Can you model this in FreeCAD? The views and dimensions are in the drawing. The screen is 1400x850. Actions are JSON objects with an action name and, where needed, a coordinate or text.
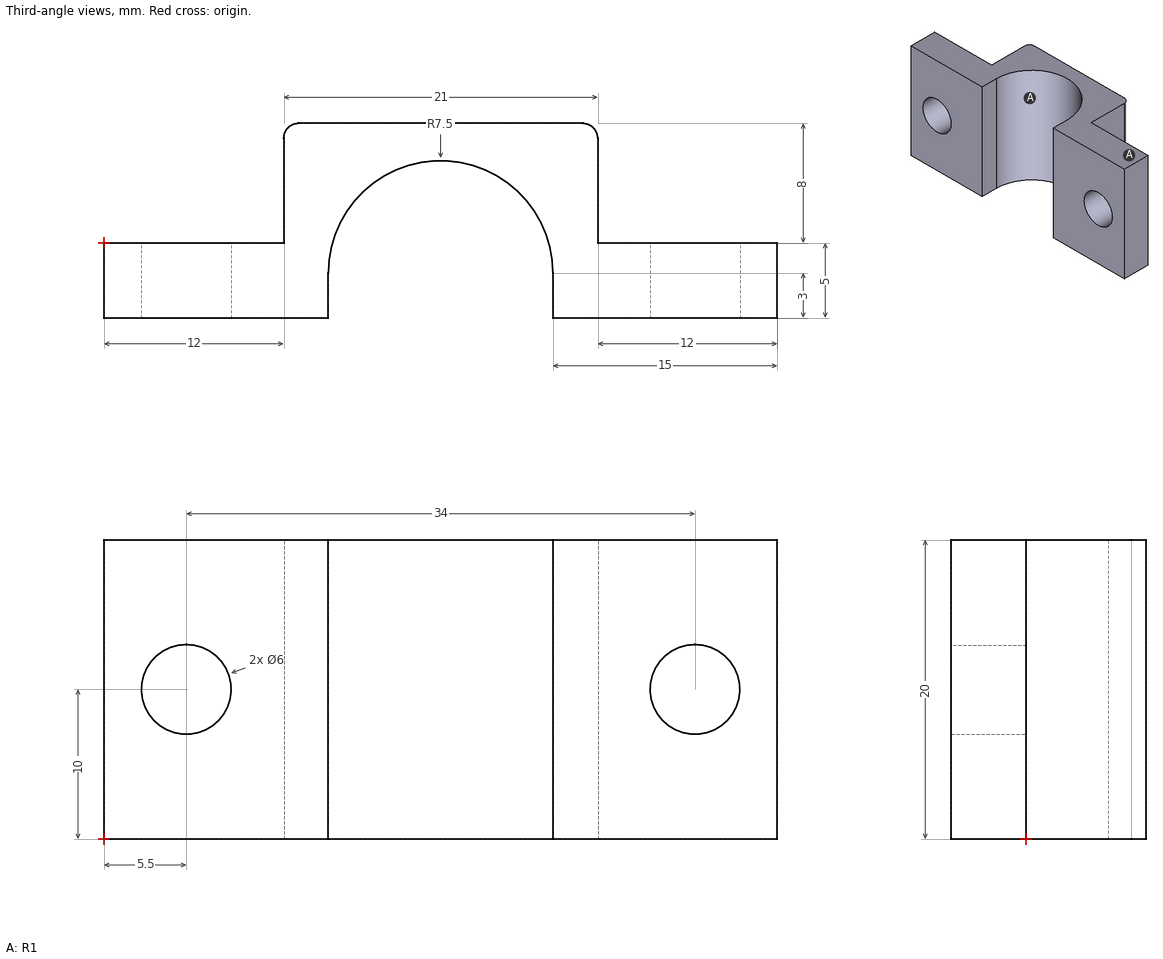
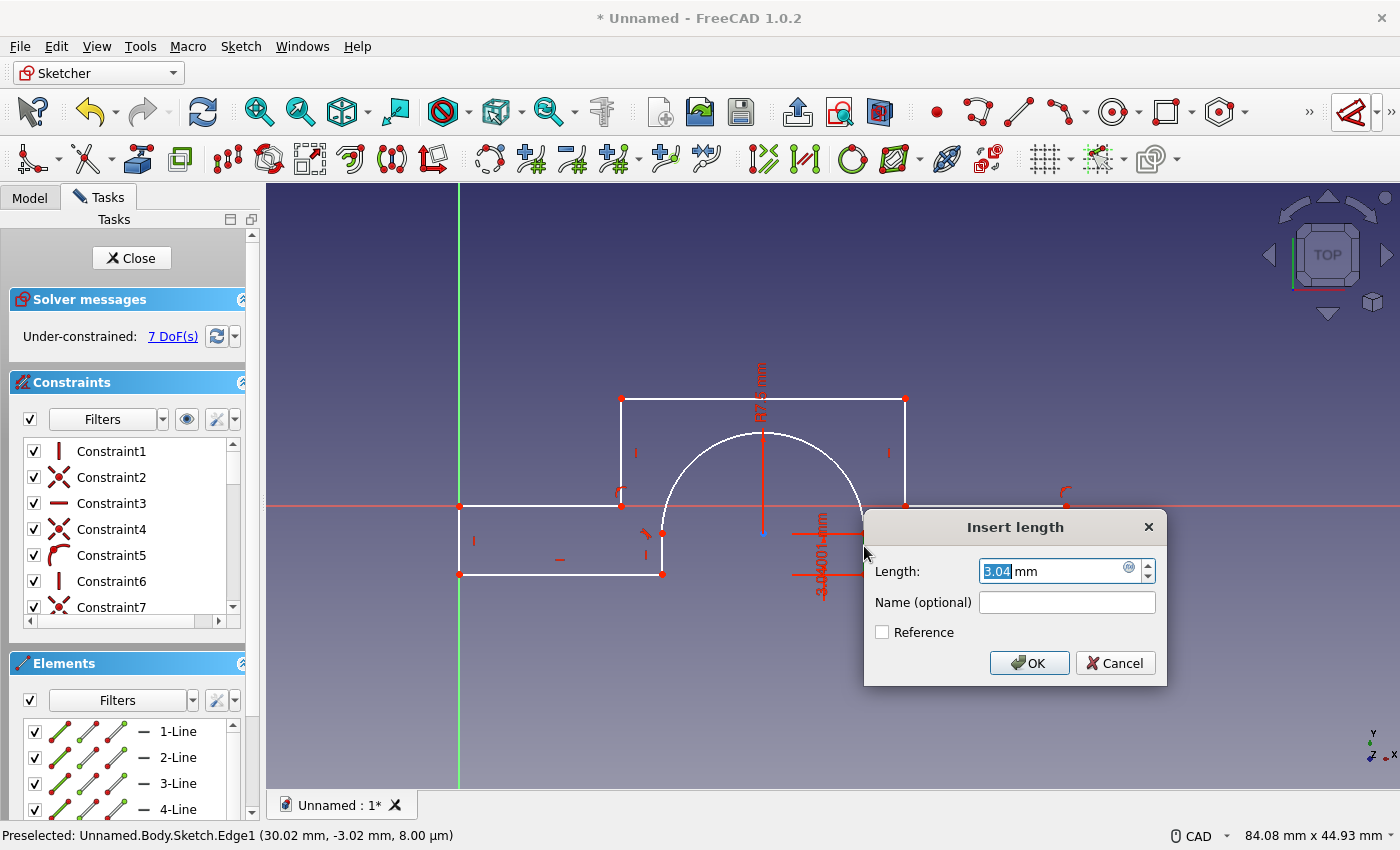
{"action": "type", "text": "3"}
{"action": "key", "text": "Return"}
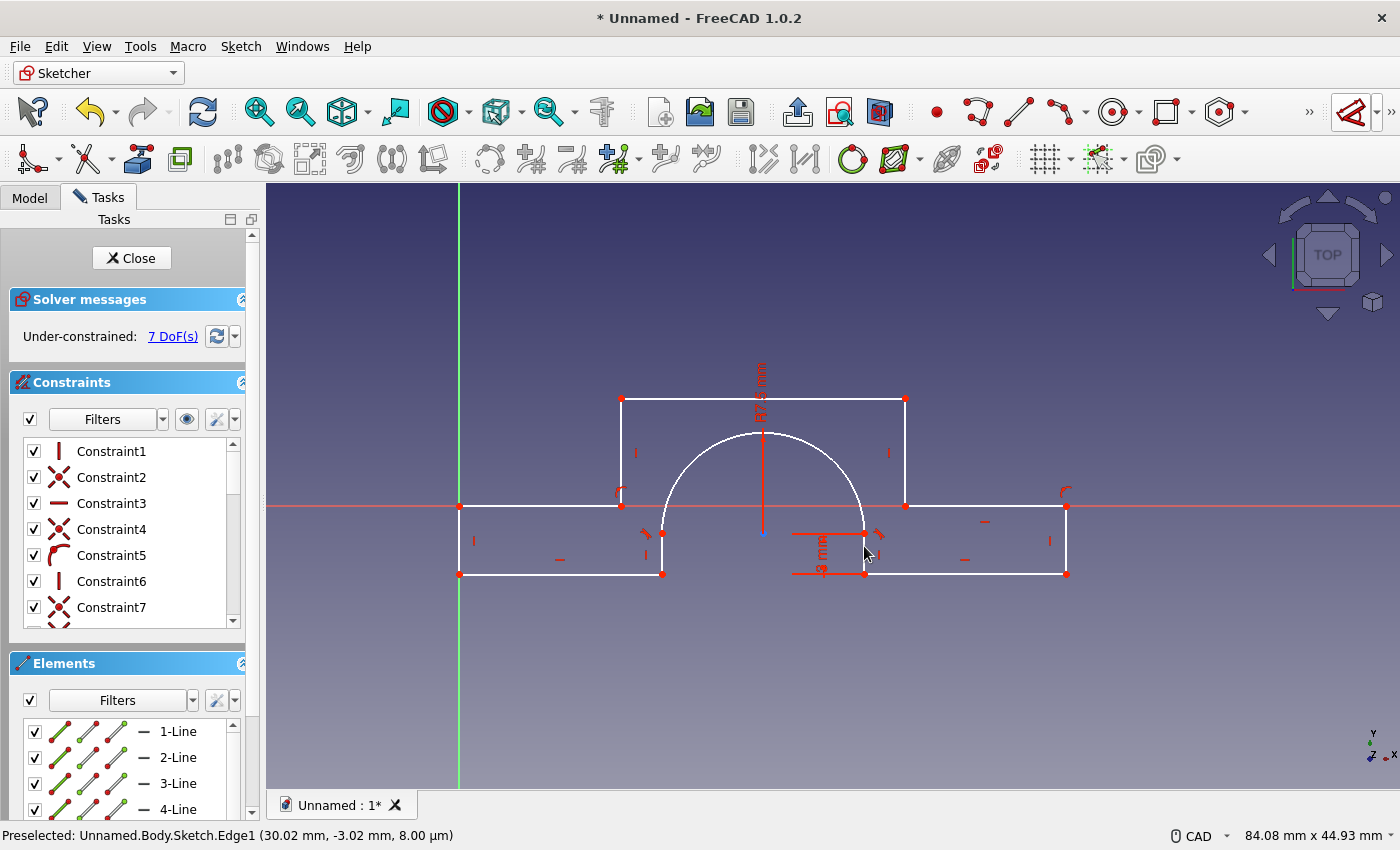
{"action": "left_click", "coordinate": [1066, 554]}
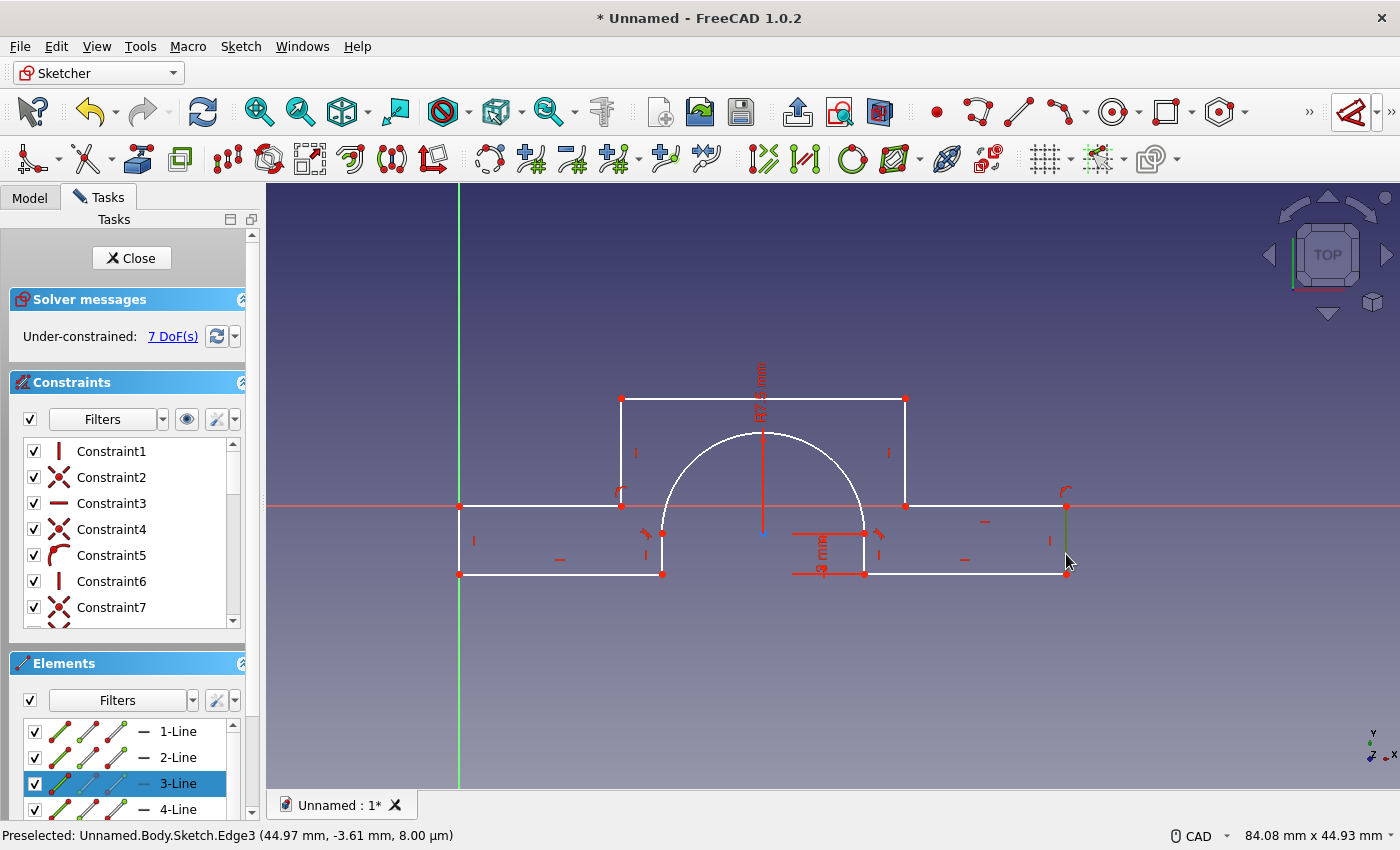
{"action": "key", "text": "i"}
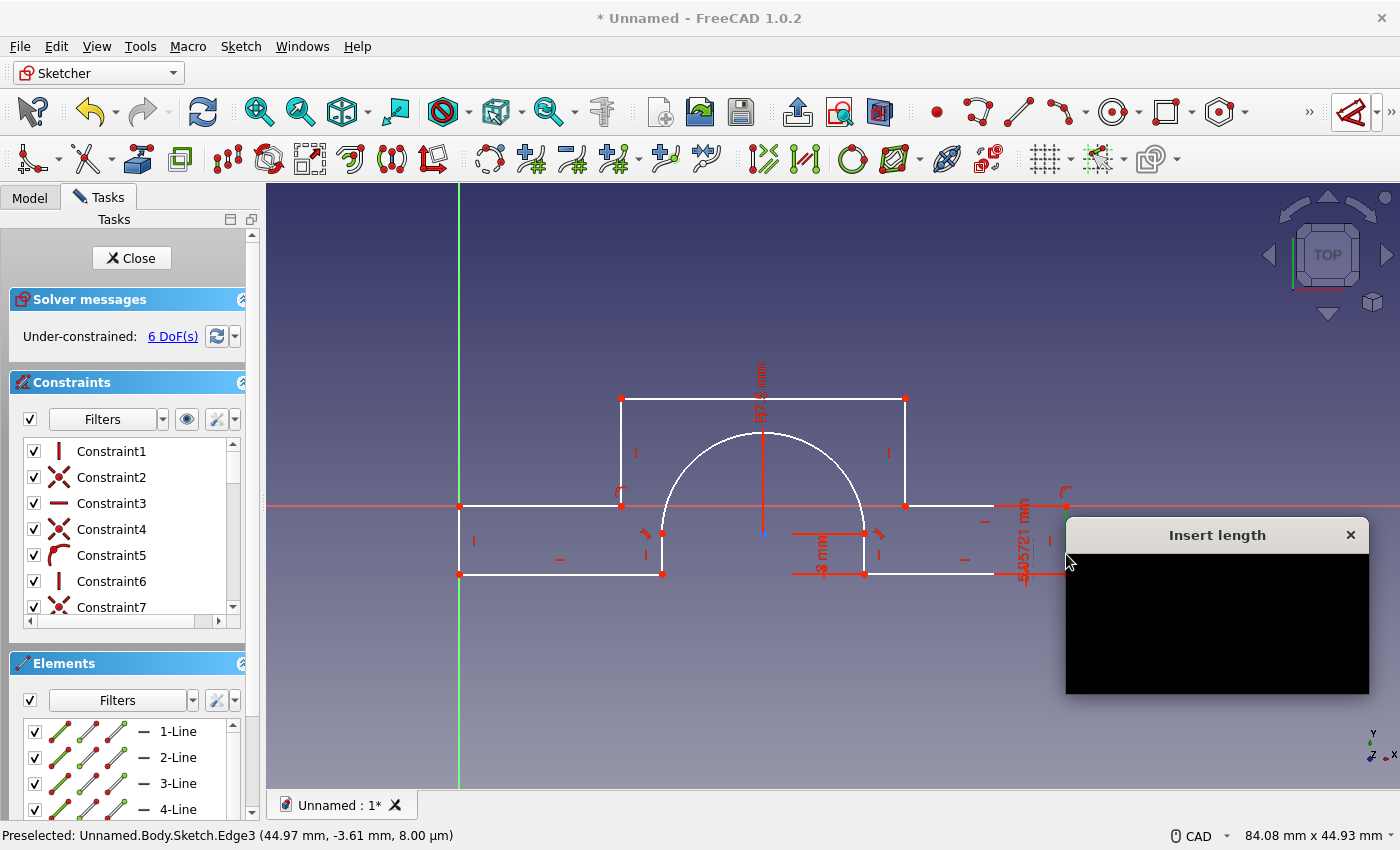
{"action": "type", "text": "5"}
{"action": "key", "text": "Return"}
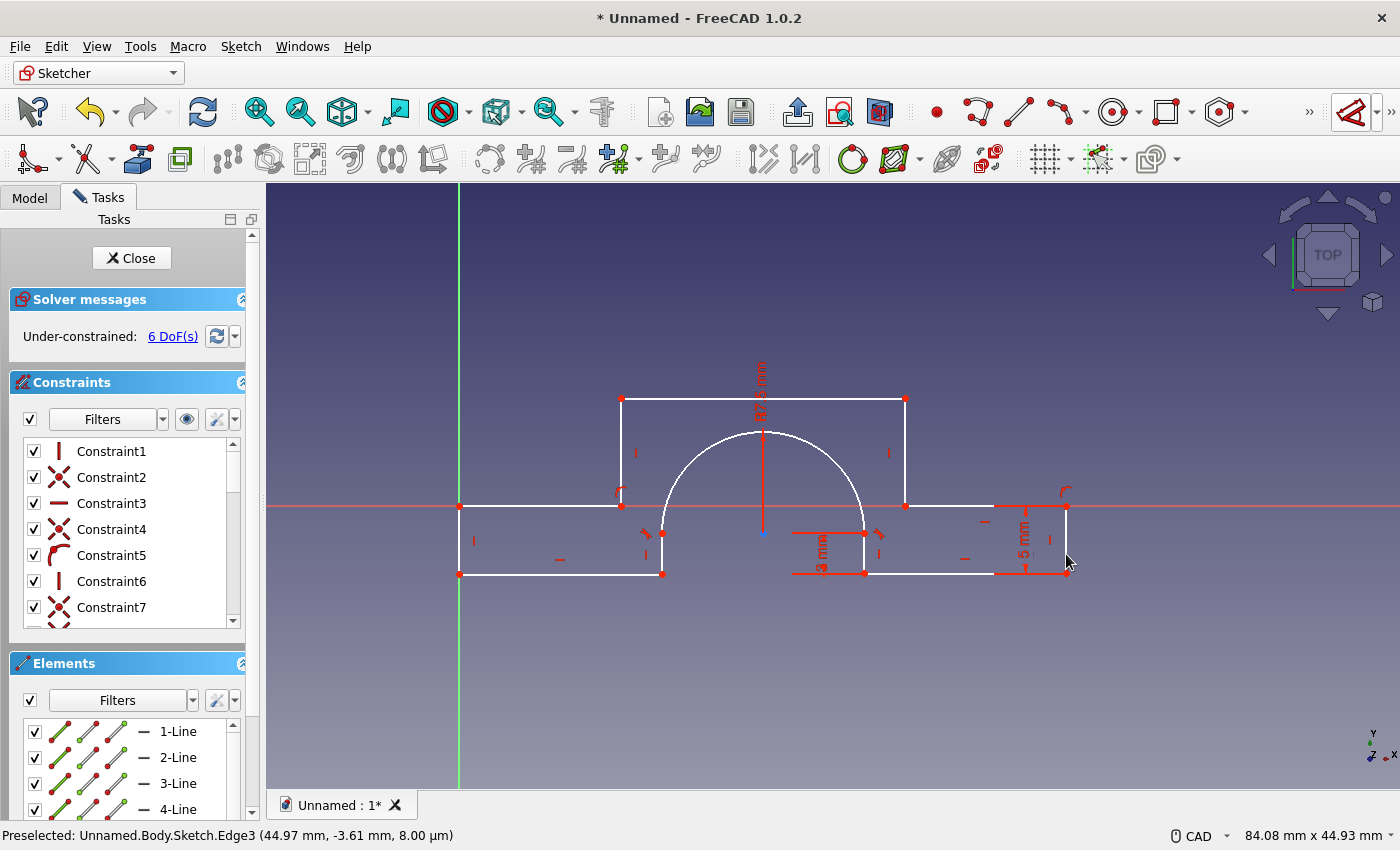
{"action": "left_click", "coordinate": [905, 474]}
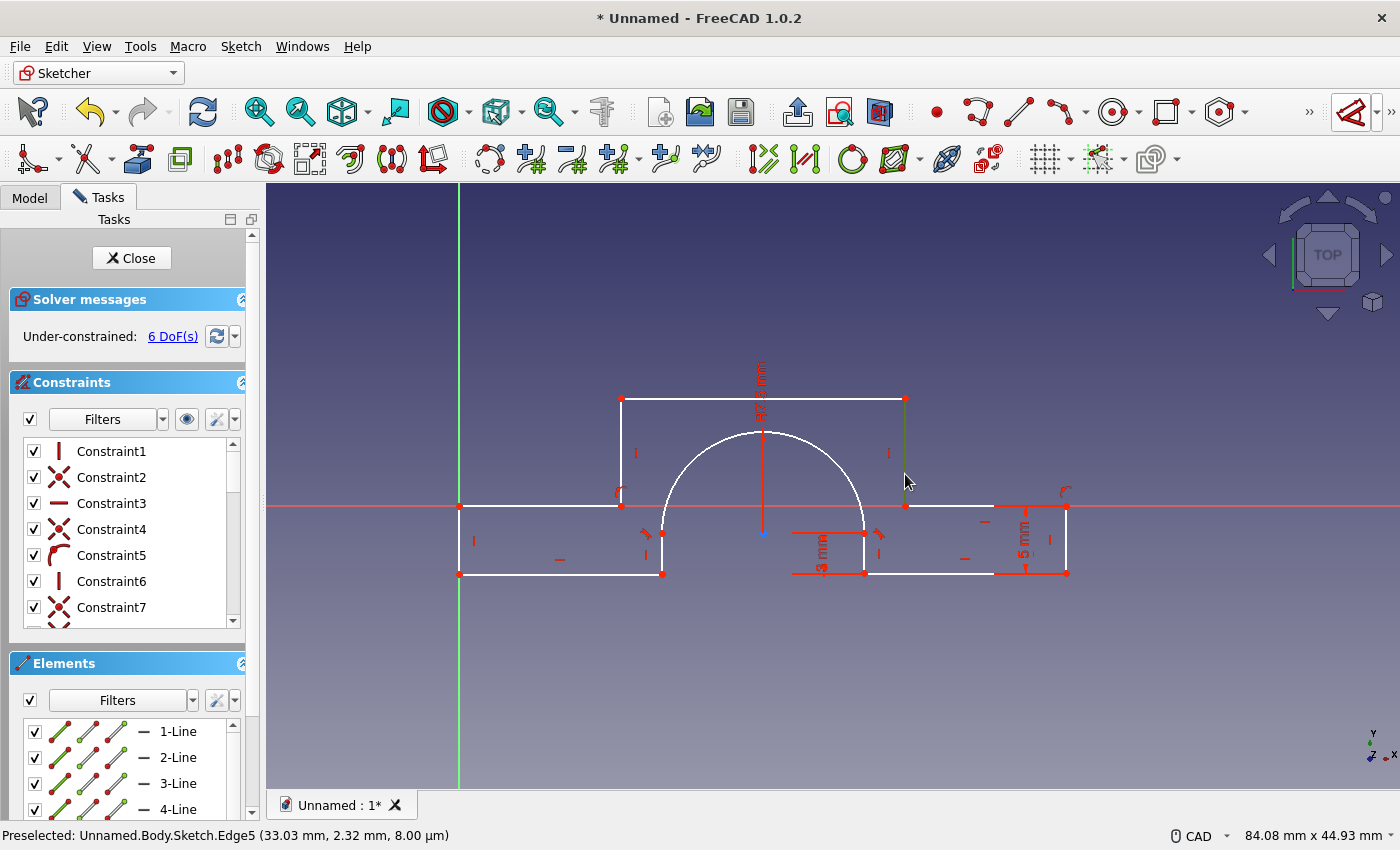
{"action": "key", "text": "i"}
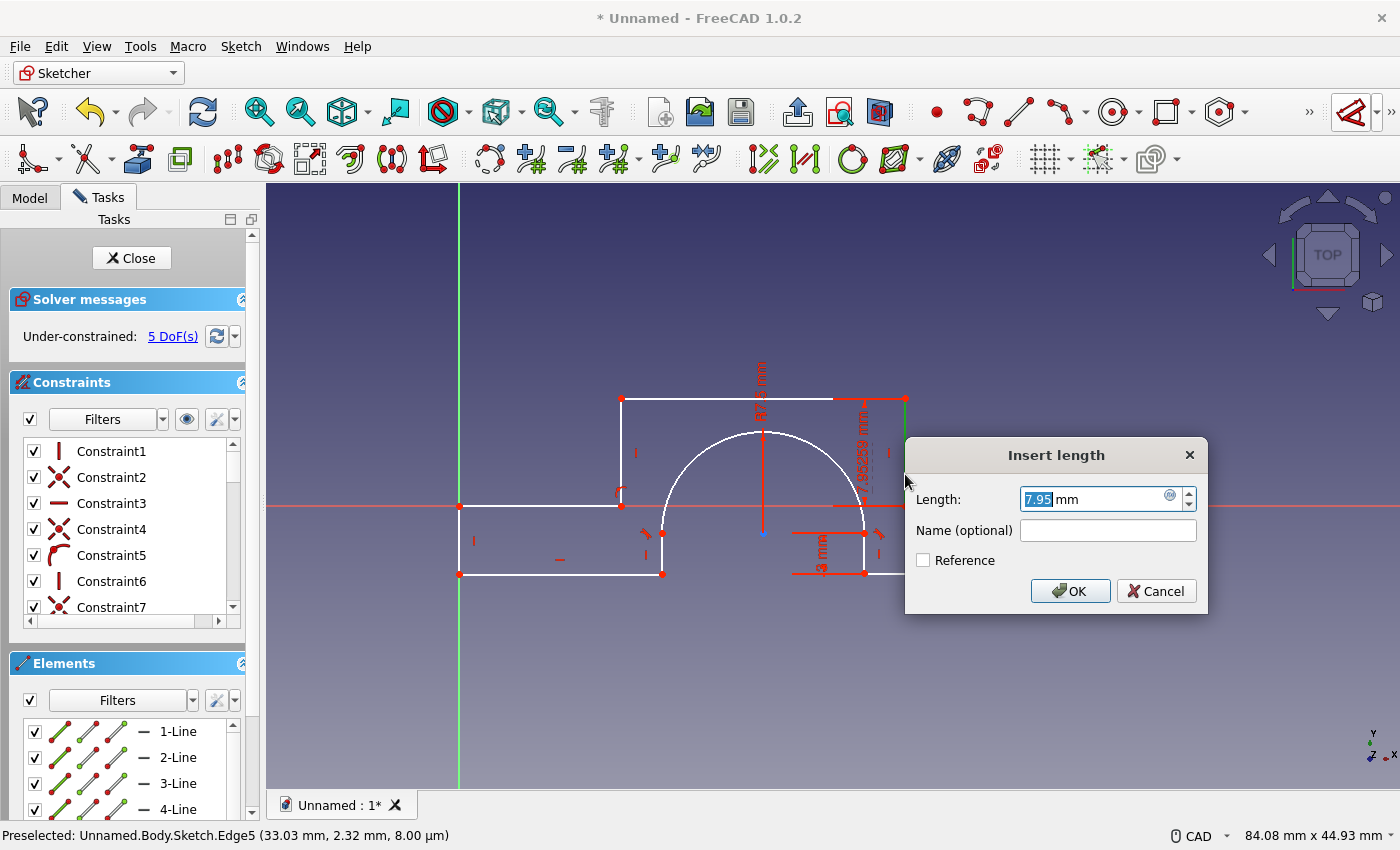
{"action": "type", "text": "8"}
{"action": "key", "text": "Return"}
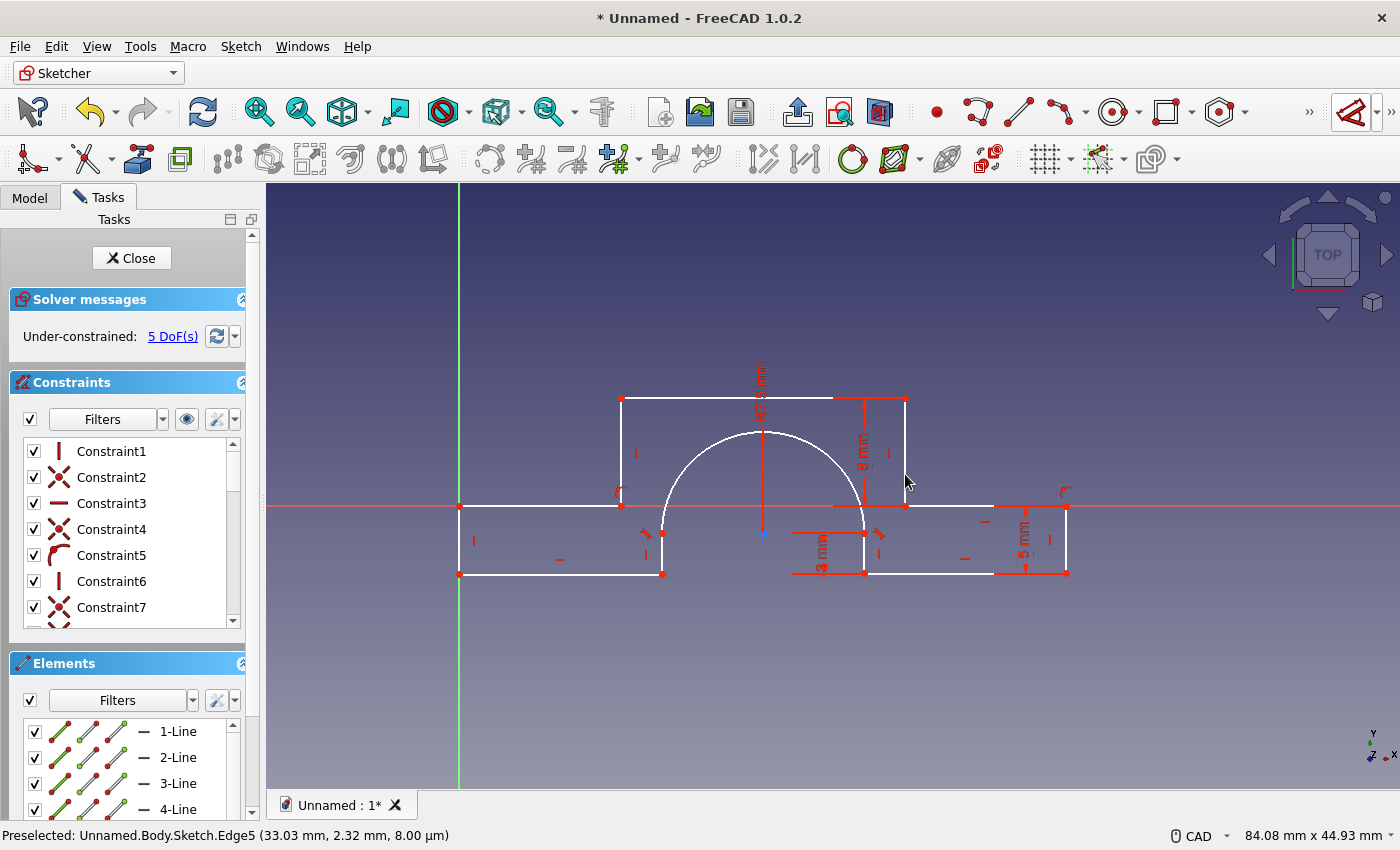
{"action": "left_click", "coordinate": [459, 527]}